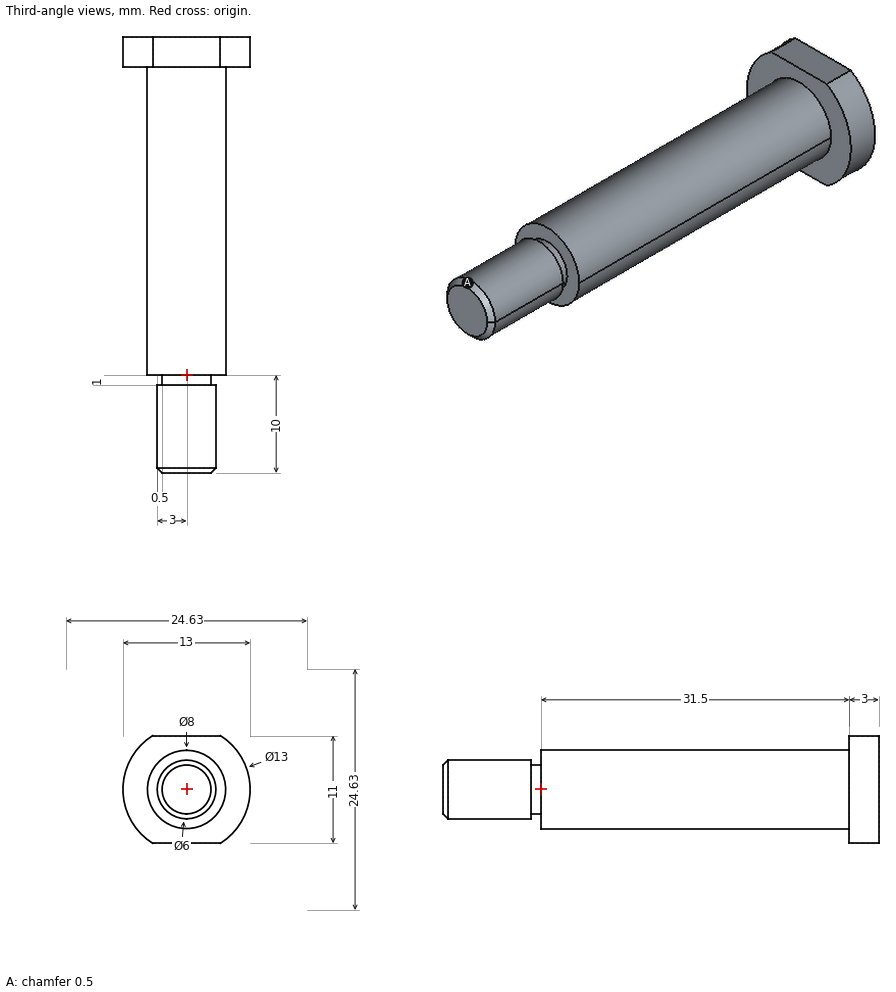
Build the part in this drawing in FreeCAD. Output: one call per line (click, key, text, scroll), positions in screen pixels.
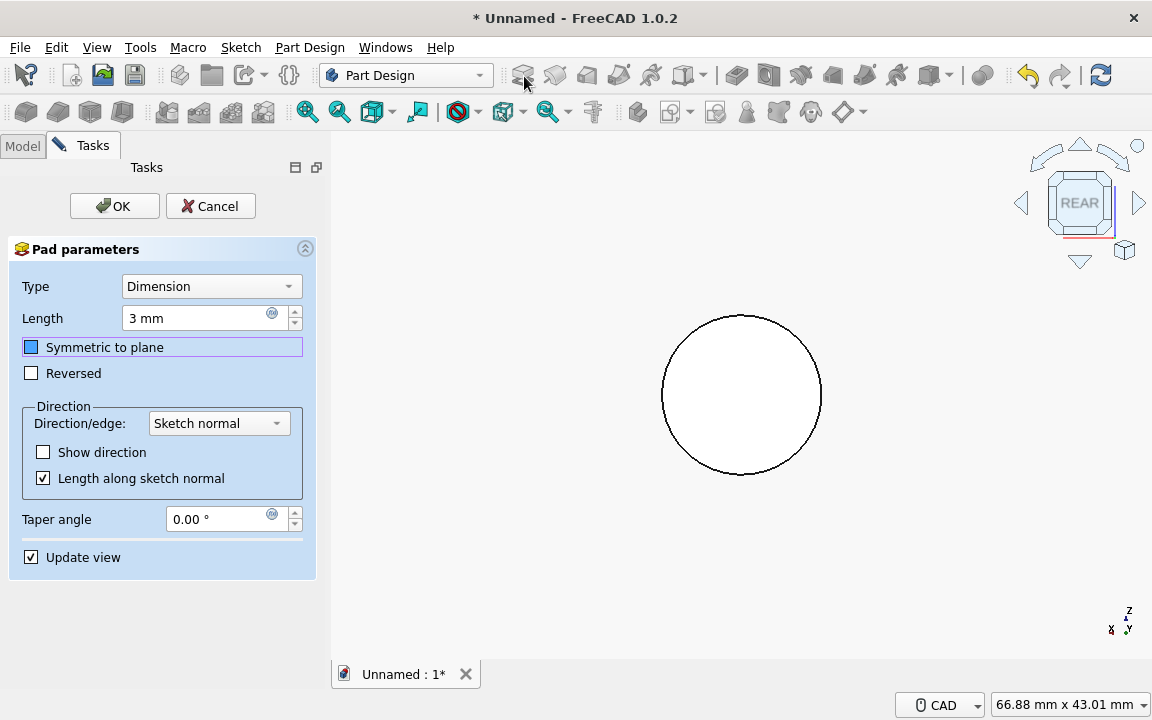
click(115, 206)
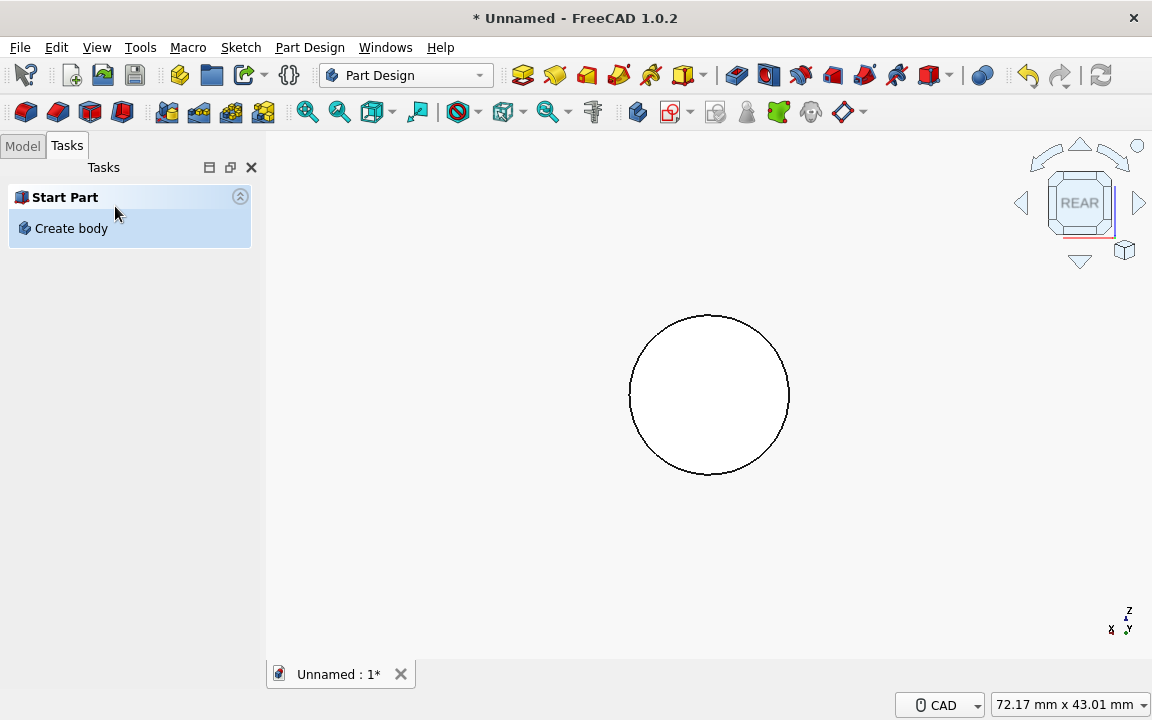
key(v)
key(f)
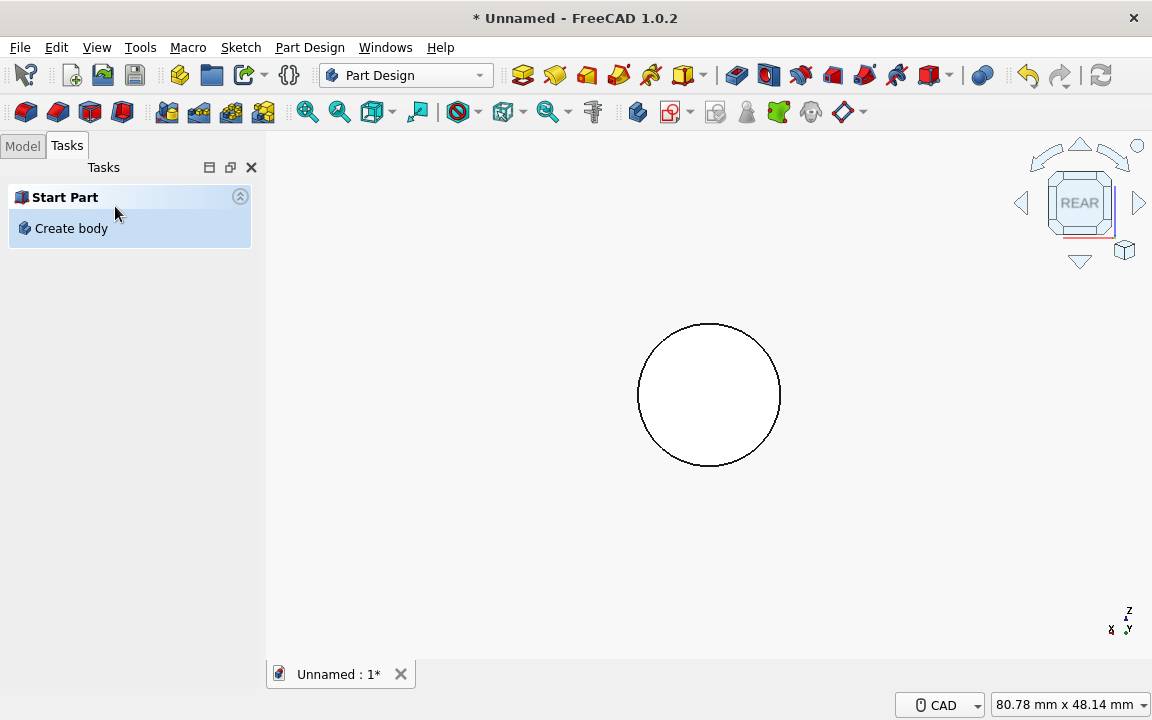
click(709, 394)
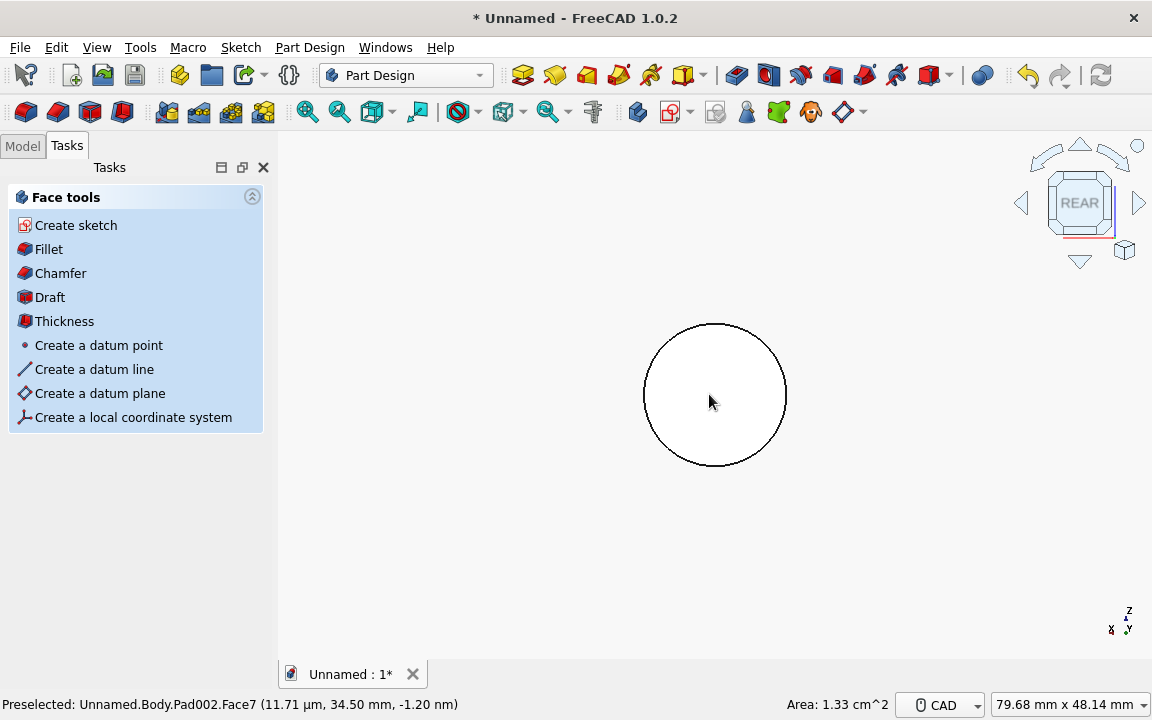
click(670, 112)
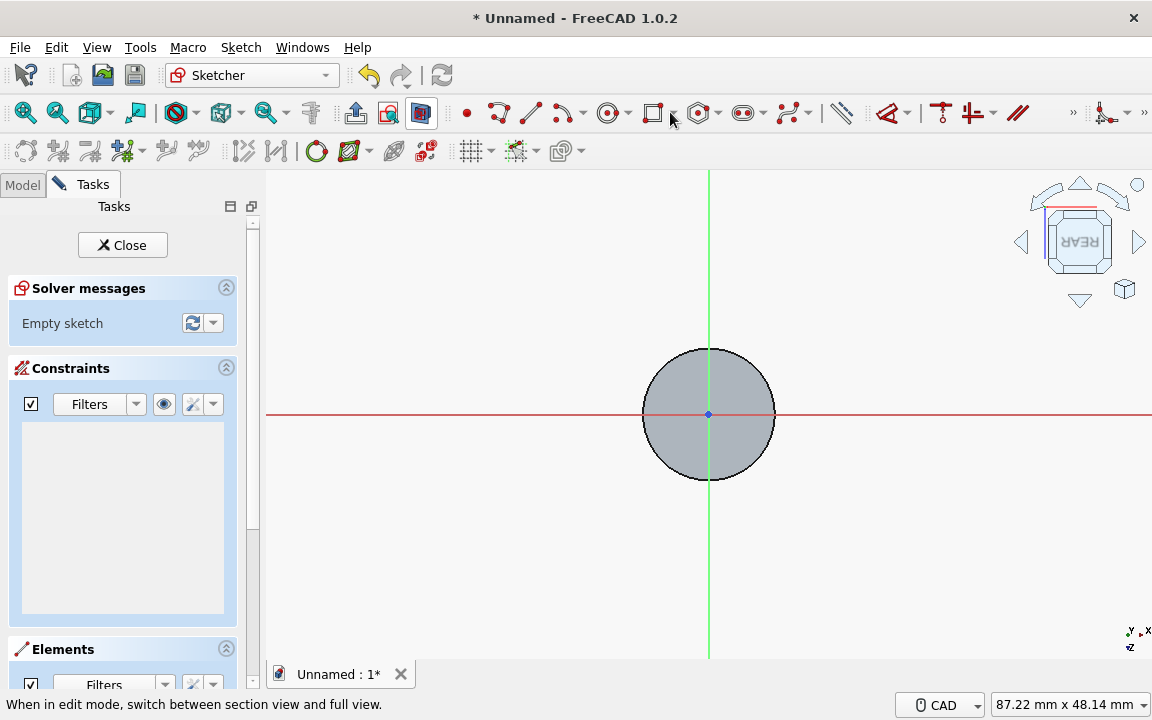
key(g)
key(v)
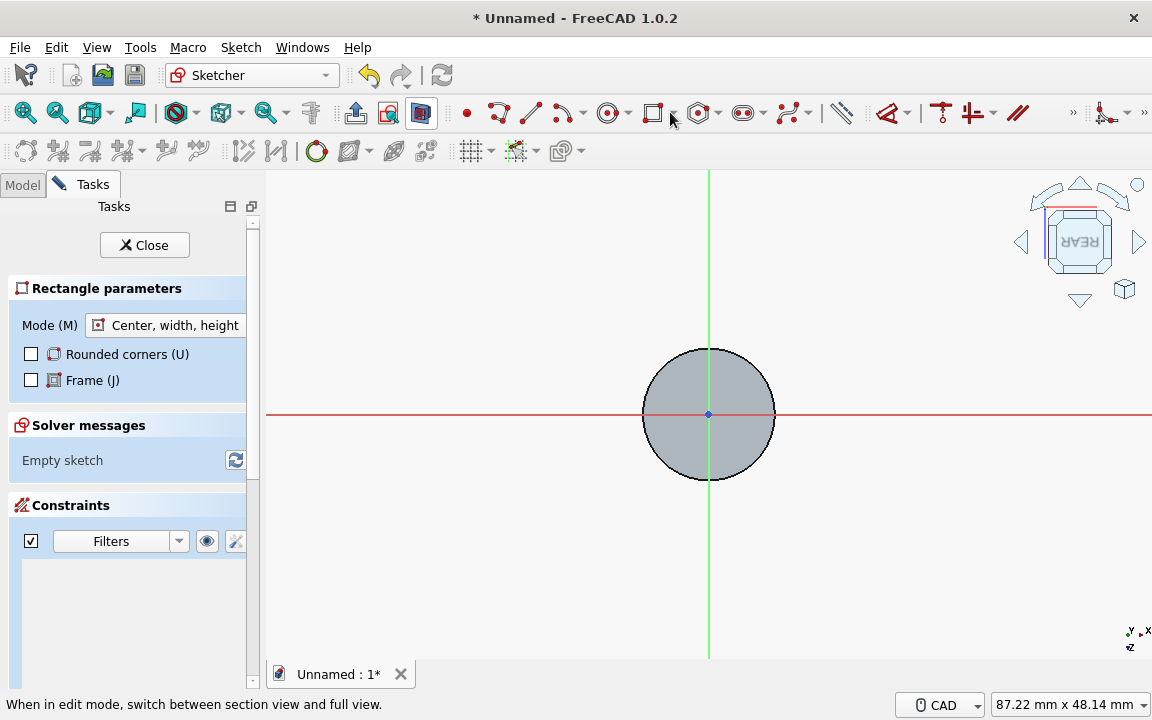
click(709, 414)
move(834, 289)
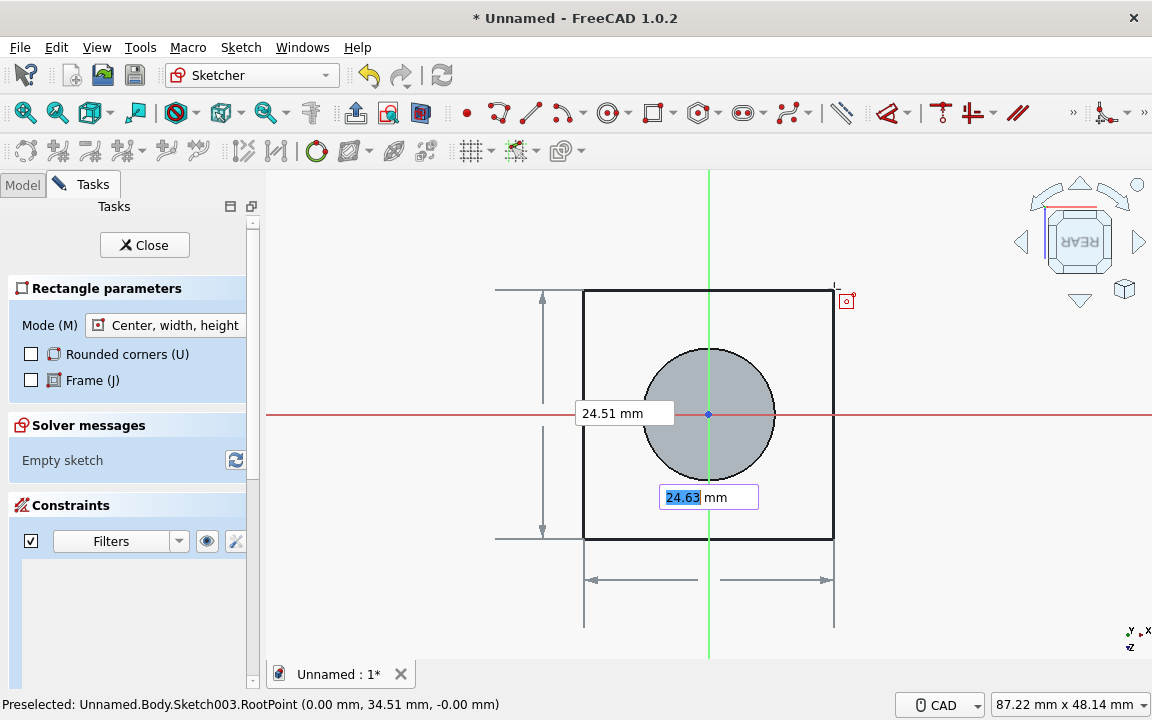
text(24.63)
key(Tab)
text(24.63)
key(Return)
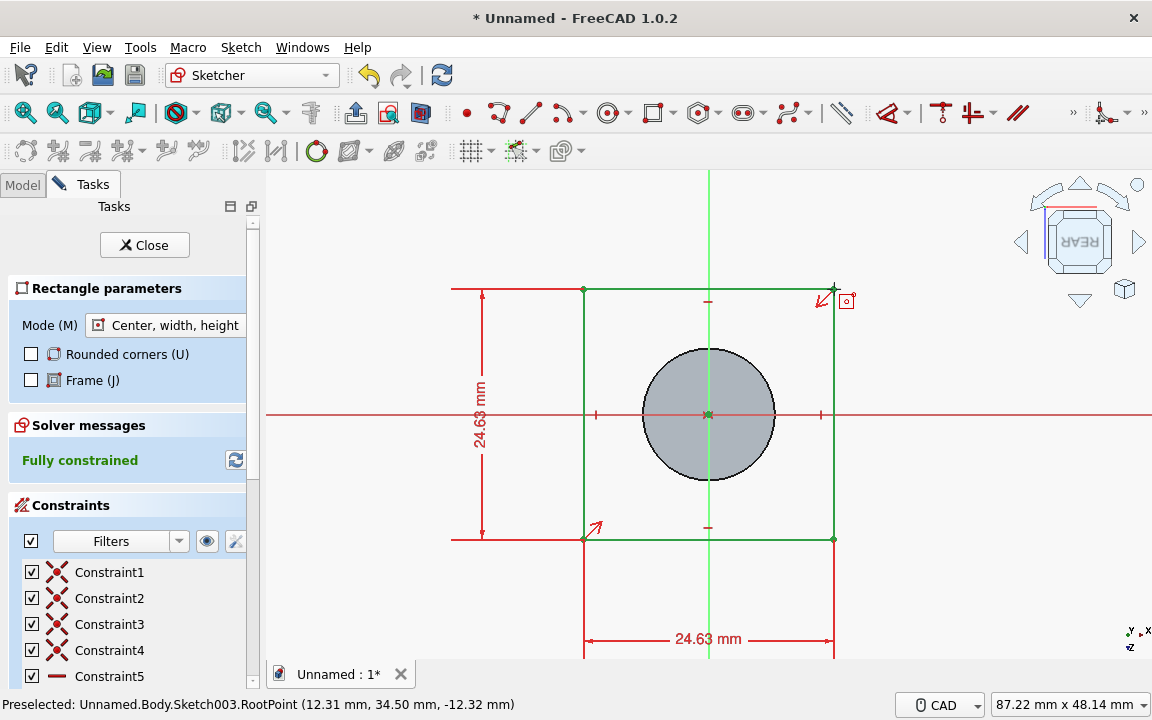
click(709, 414)
move(775, 359)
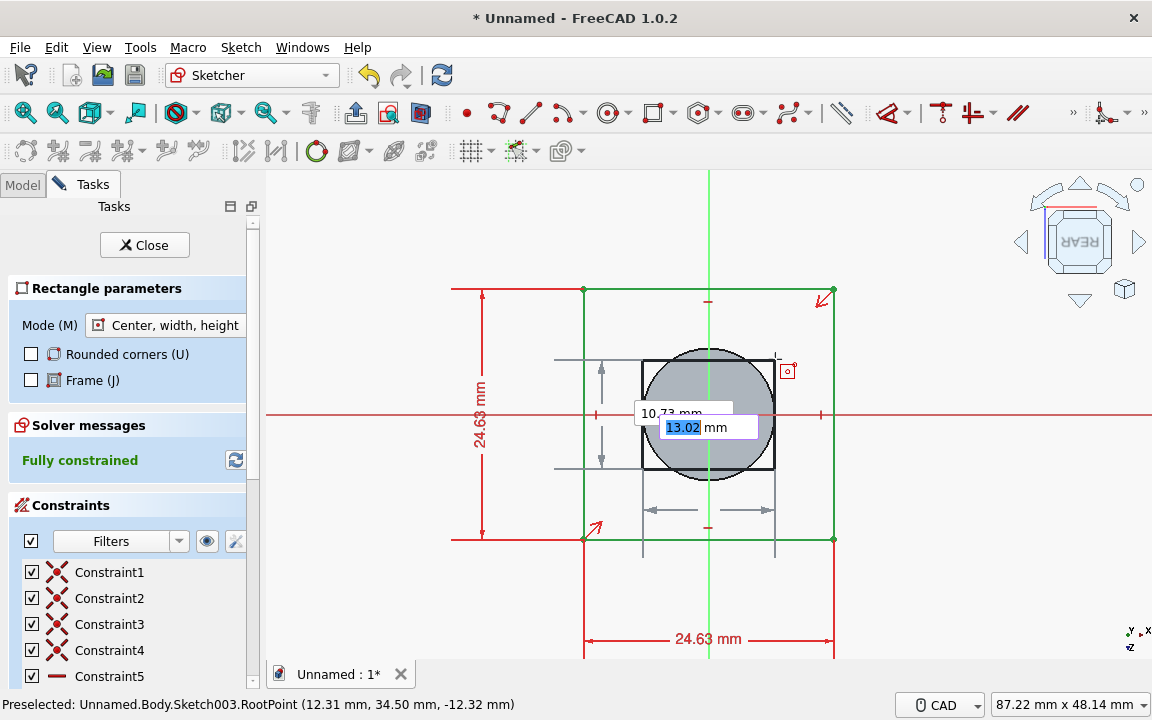
text(13)
key(Tab)
text(11)
key(Return)
key(Escape)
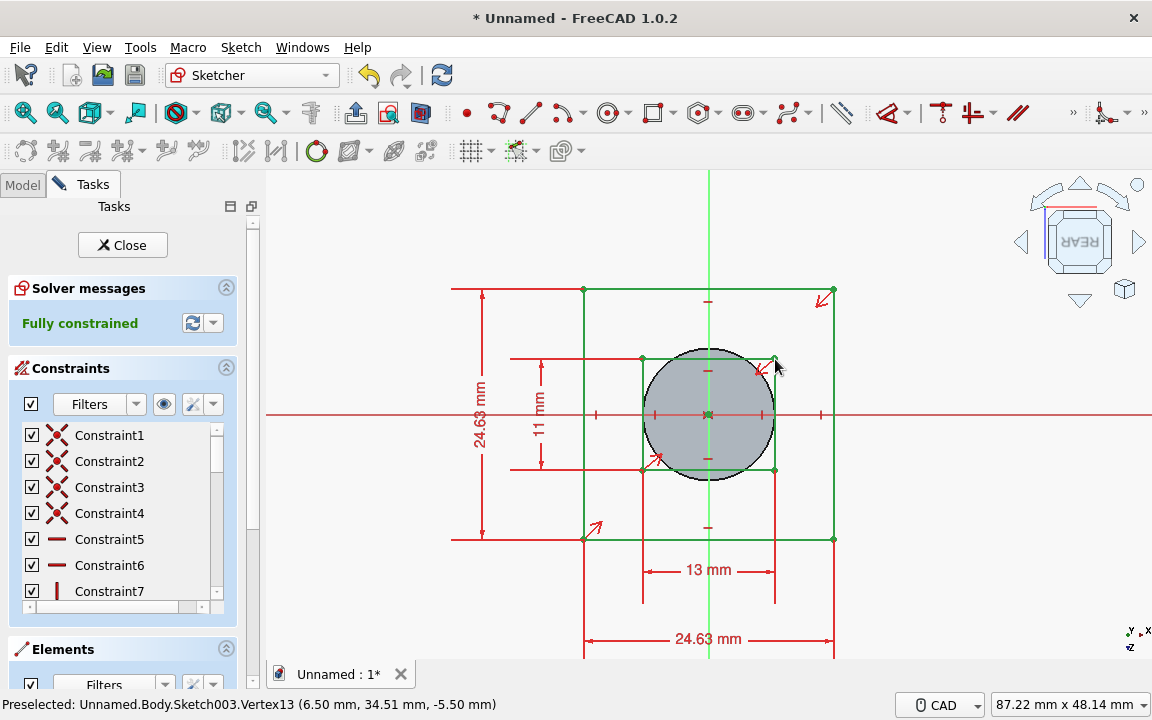
click(123, 245)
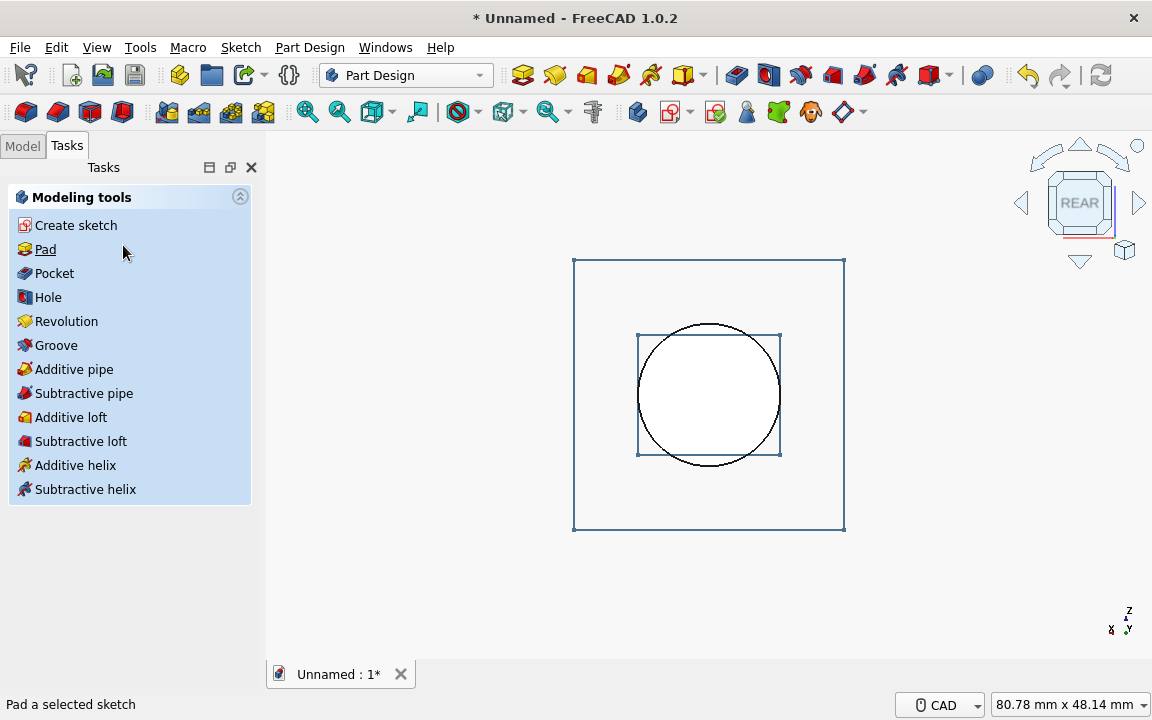
click(738, 76)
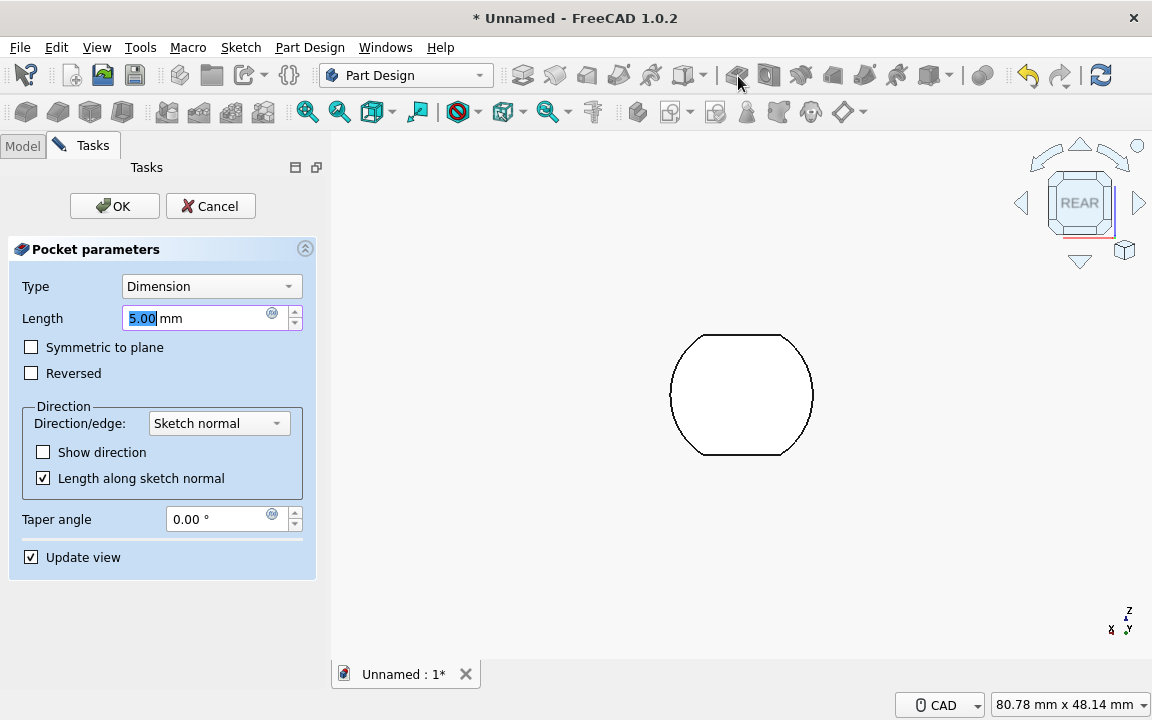
click(212, 286)